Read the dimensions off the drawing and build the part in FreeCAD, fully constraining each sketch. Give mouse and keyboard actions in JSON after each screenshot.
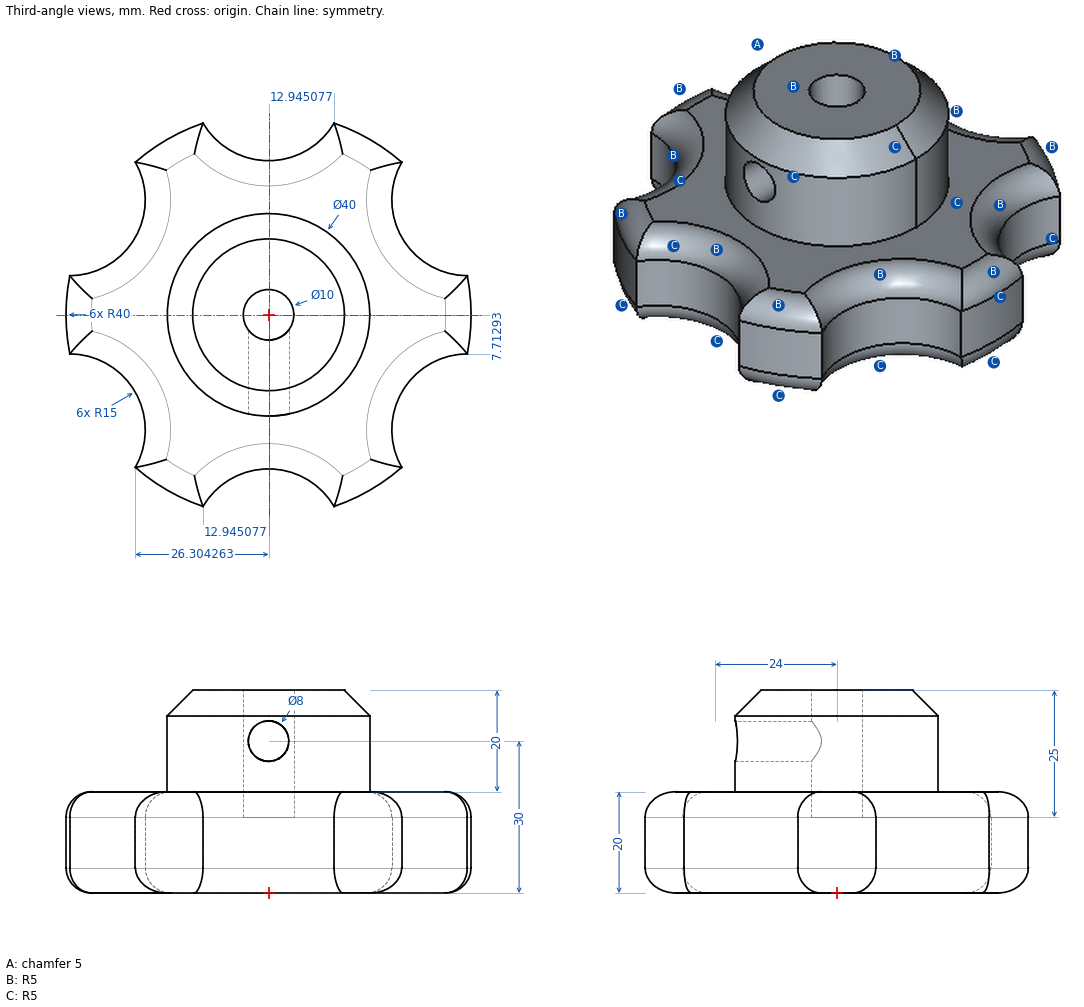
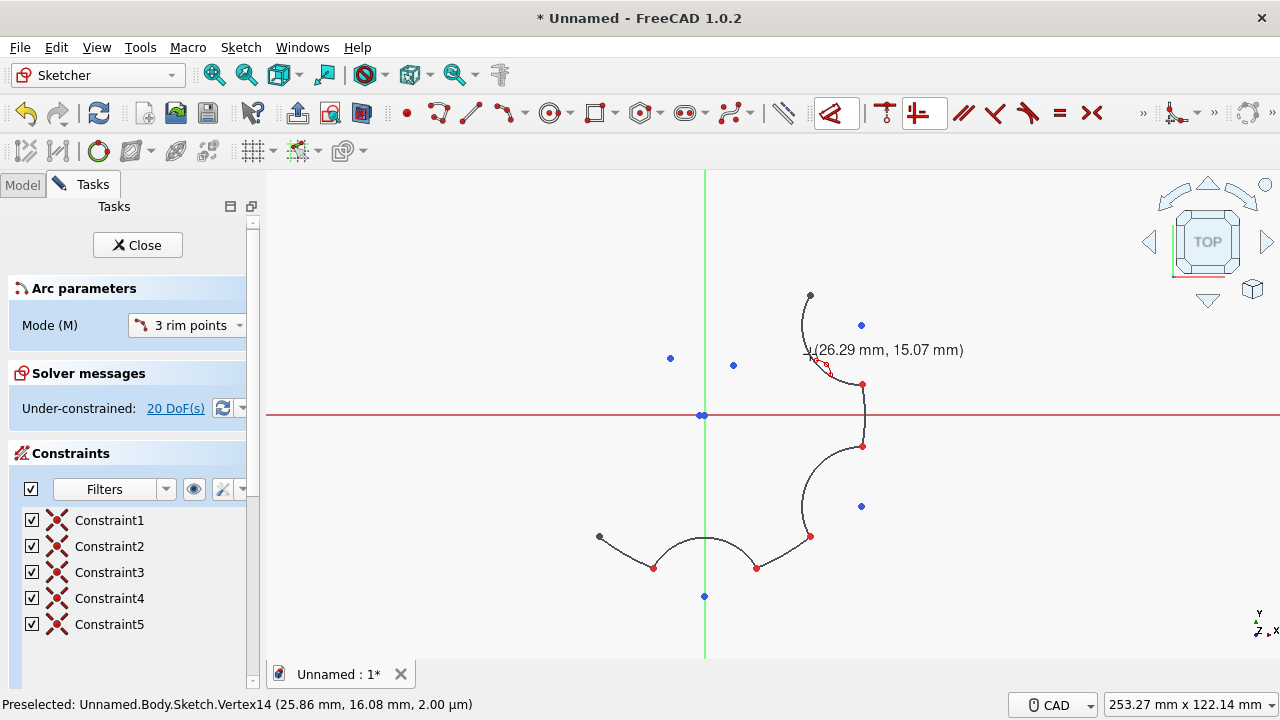
{"action": "left_click", "coordinate": [810, 296]}
{"action": "left_click", "coordinate": [757, 264]}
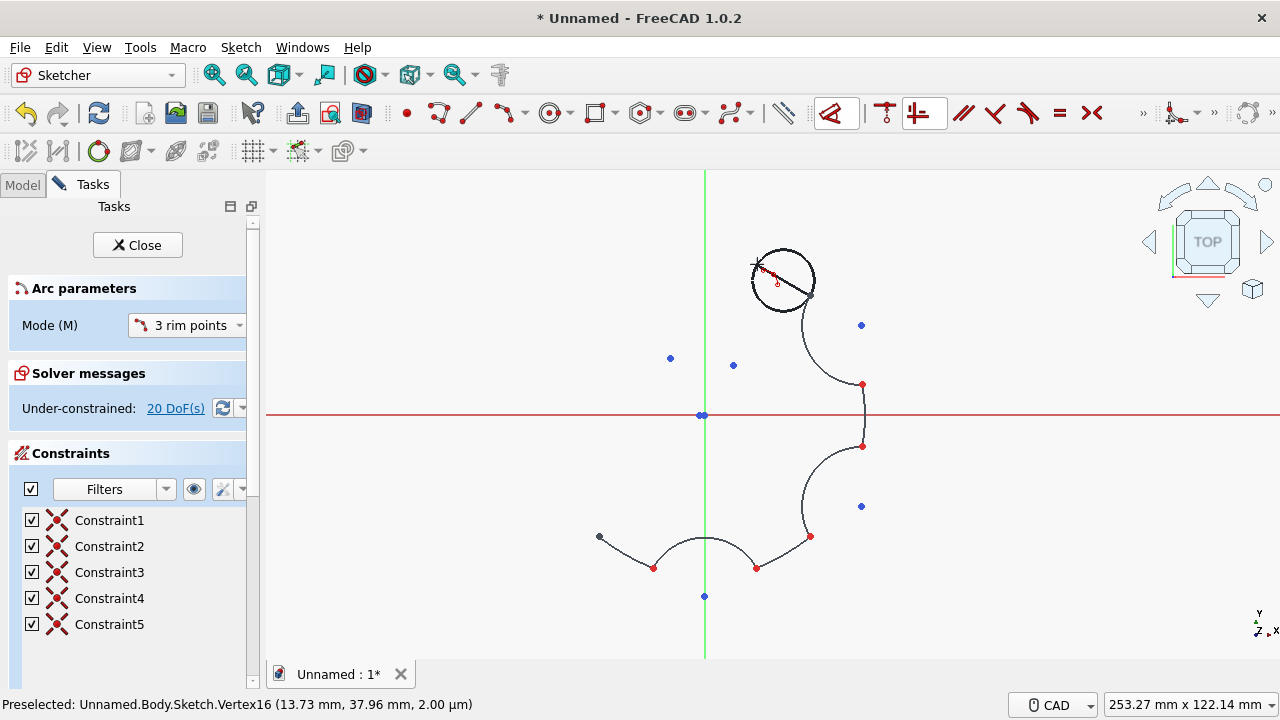
{"action": "scroll", "coordinate": [785, 277], "scroll_direction": "up", "scroll_amount": 9}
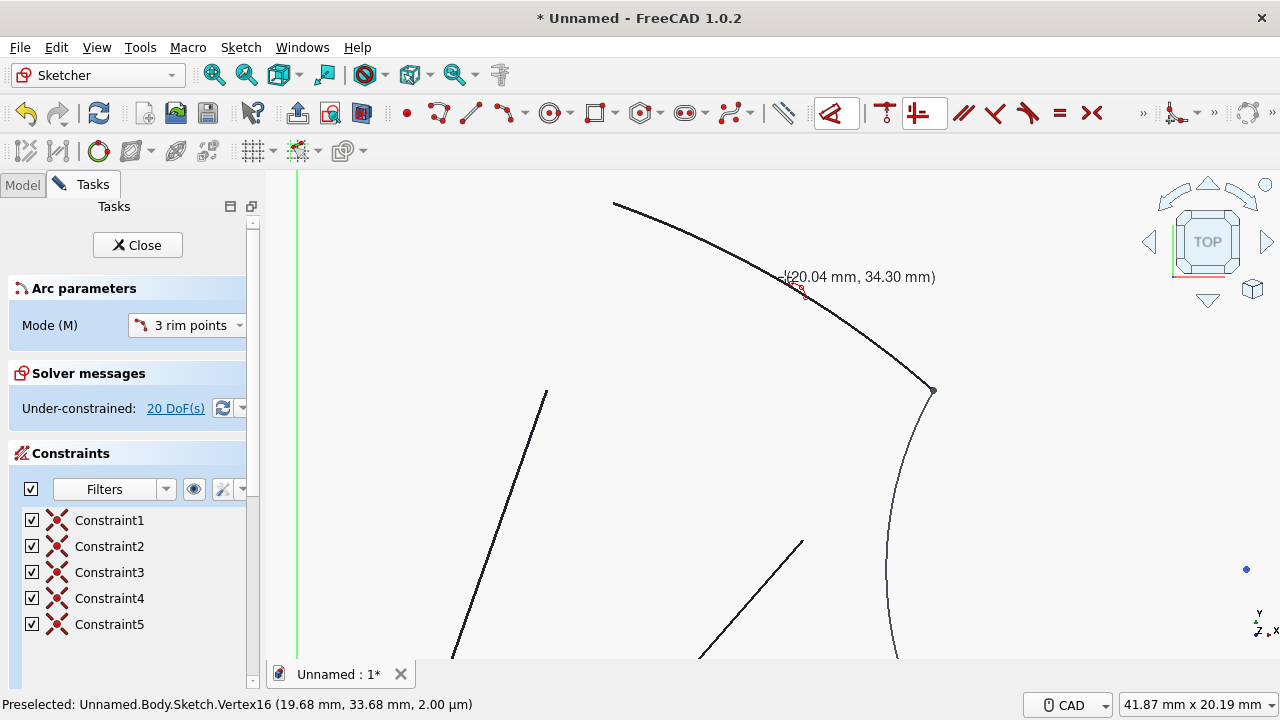
{"action": "left_click", "coordinate": [781, 274]}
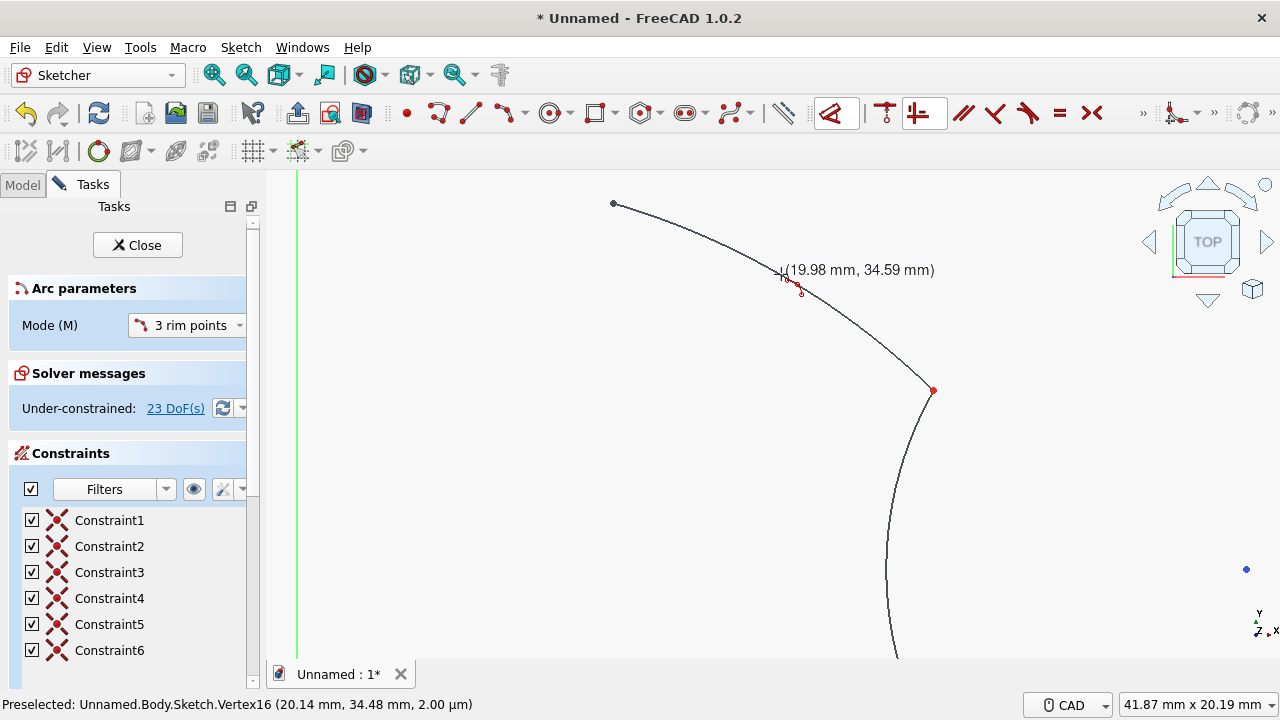
{"action": "scroll", "coordinate": [785, 276], "scroll_direction": "down", "scroll_amount": 9}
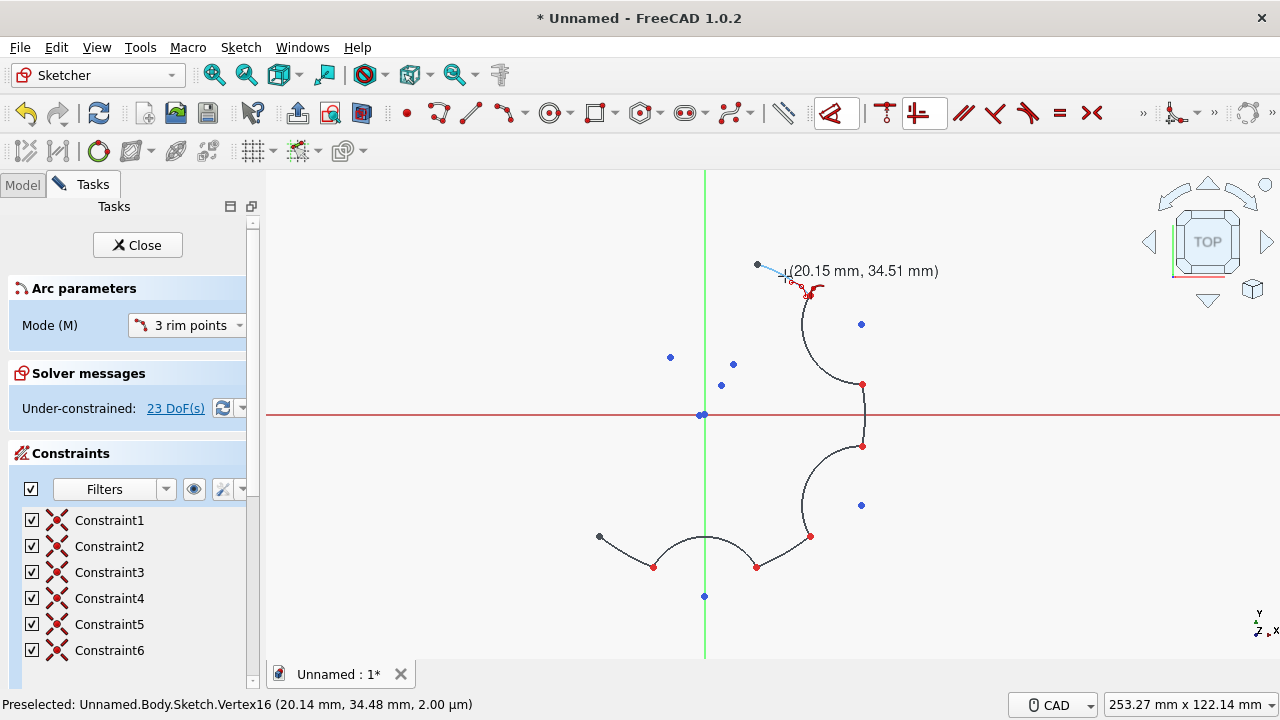
{"action": "left_click", "coordinate": [757, 264]}
{"action": "left_click", "coordinate": [653, 263]}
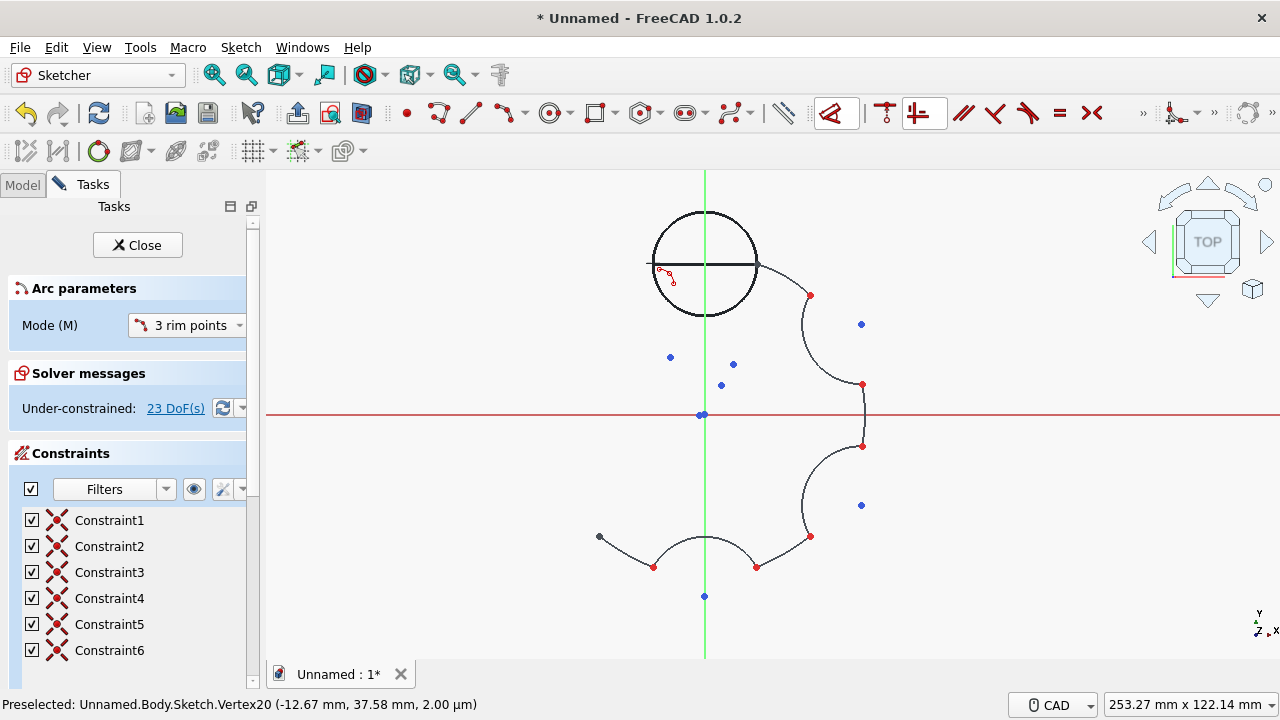
{"action": "scroll", "coordinate": [692, 291], "scroll_direction": "up", "scroll_amount": 2}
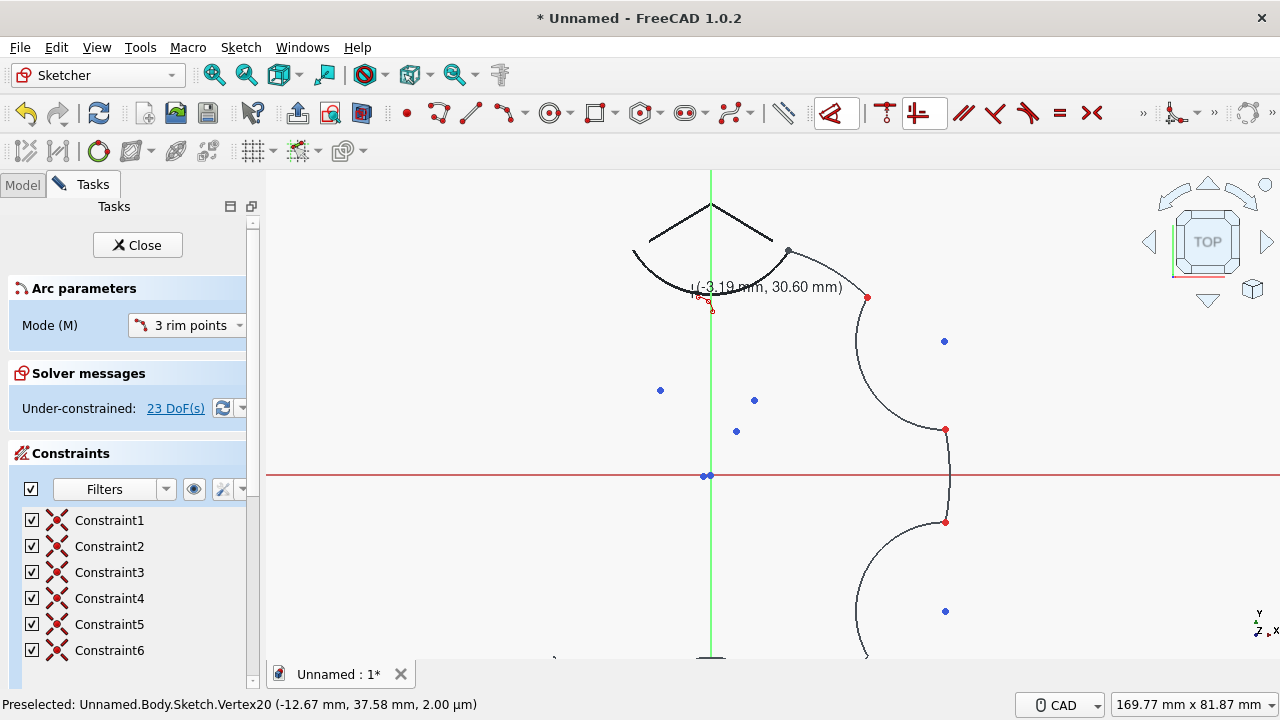
{"action": "left_click", "coordinate": [692, 291]}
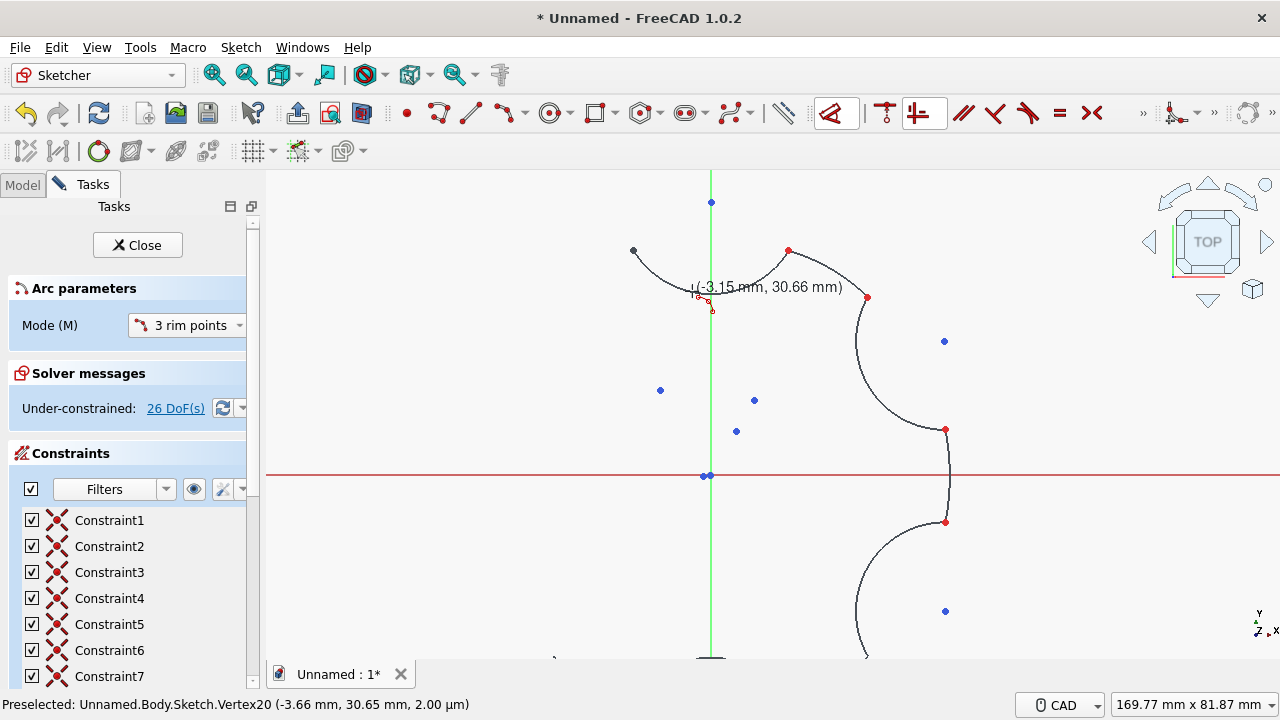
{"action": "left_click", "coordinate": [634, 251]}
{"action": "left_click", "coordinate": [554, 295]}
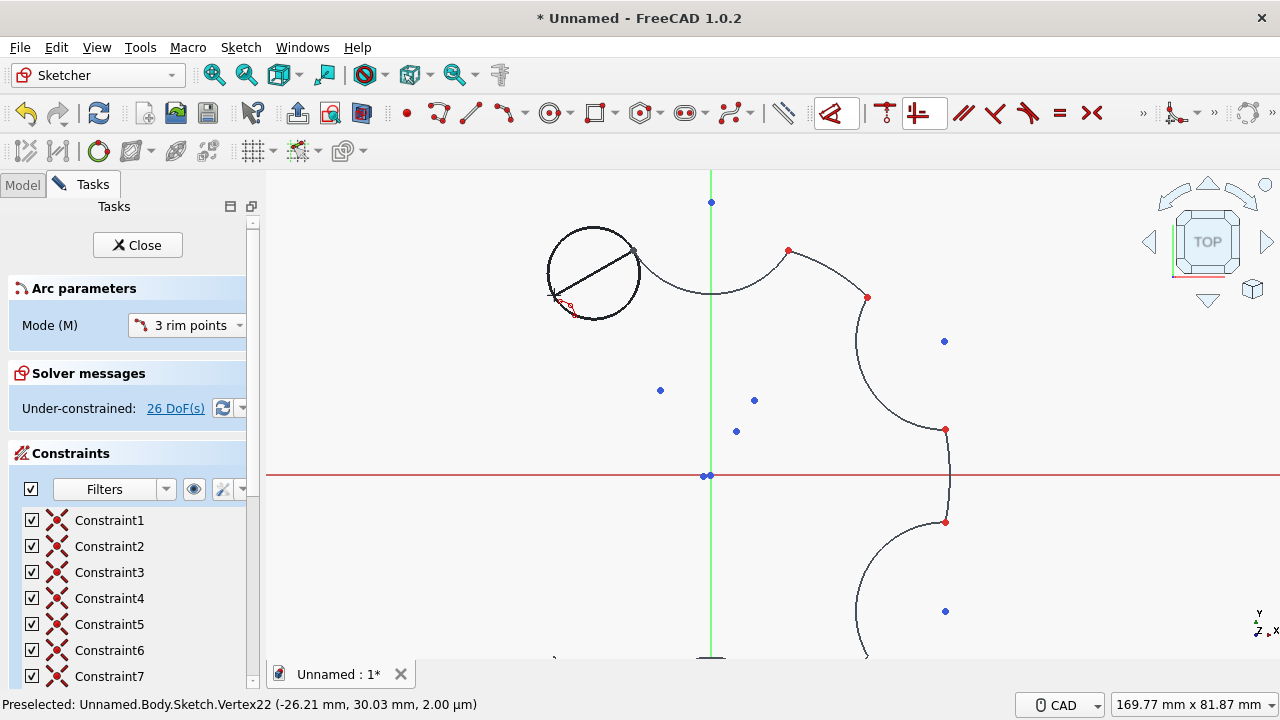
{"action": "scroll", "coordinate": [591, 268], "scroll_direction": "up", "scroll_amount": 7}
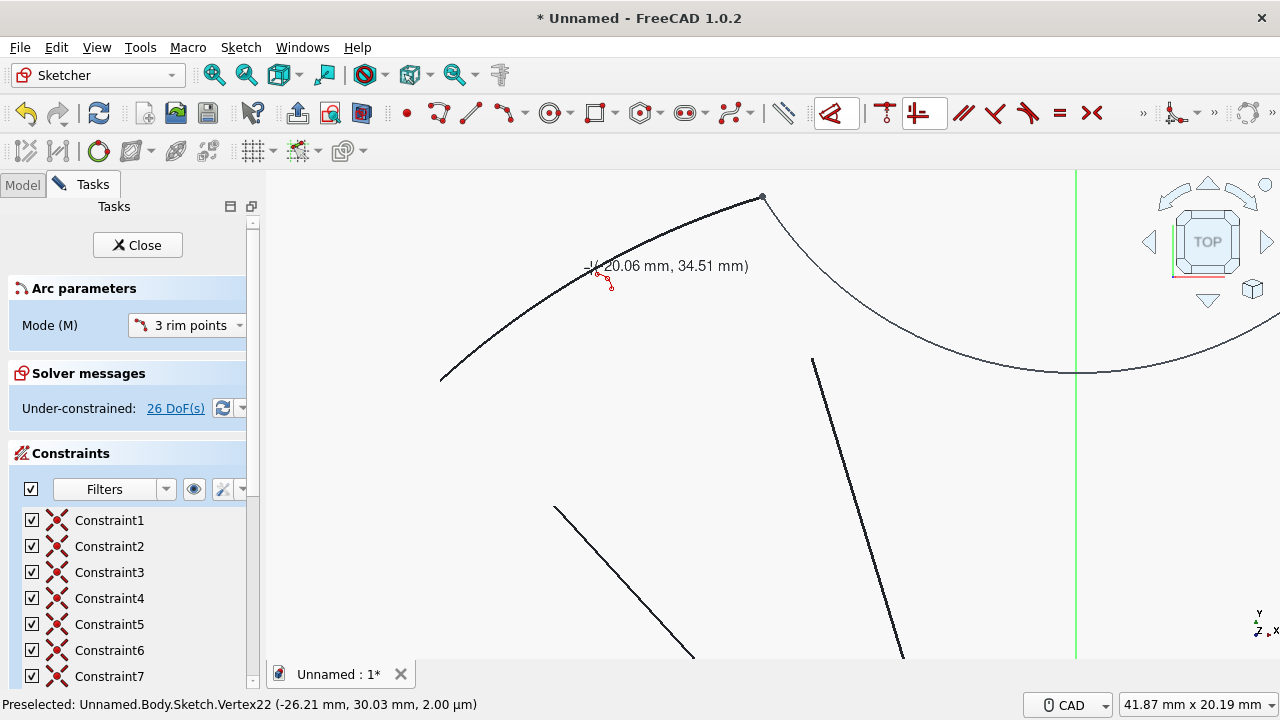
{"action": "left_click", "coordinate": [592, 268]}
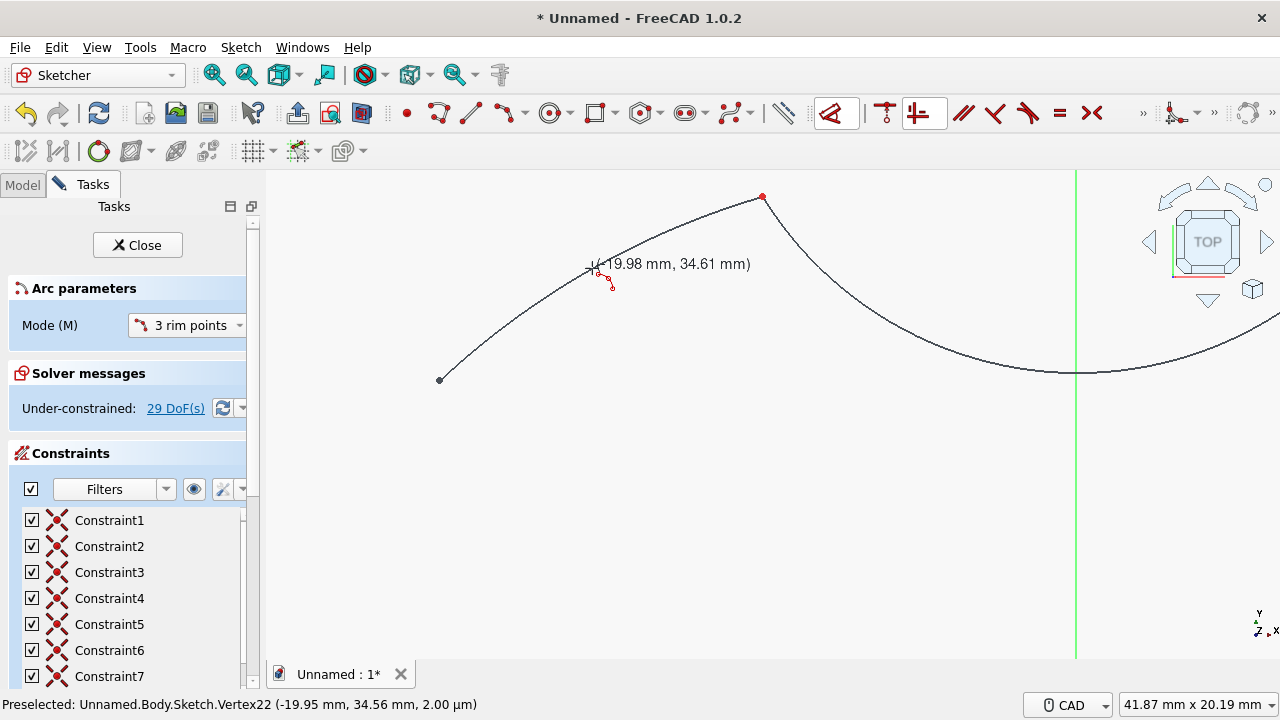
{"action": "scroll", "coordinate": [631, 277], "scroll_direction": "down", "scroll_amount": 9}